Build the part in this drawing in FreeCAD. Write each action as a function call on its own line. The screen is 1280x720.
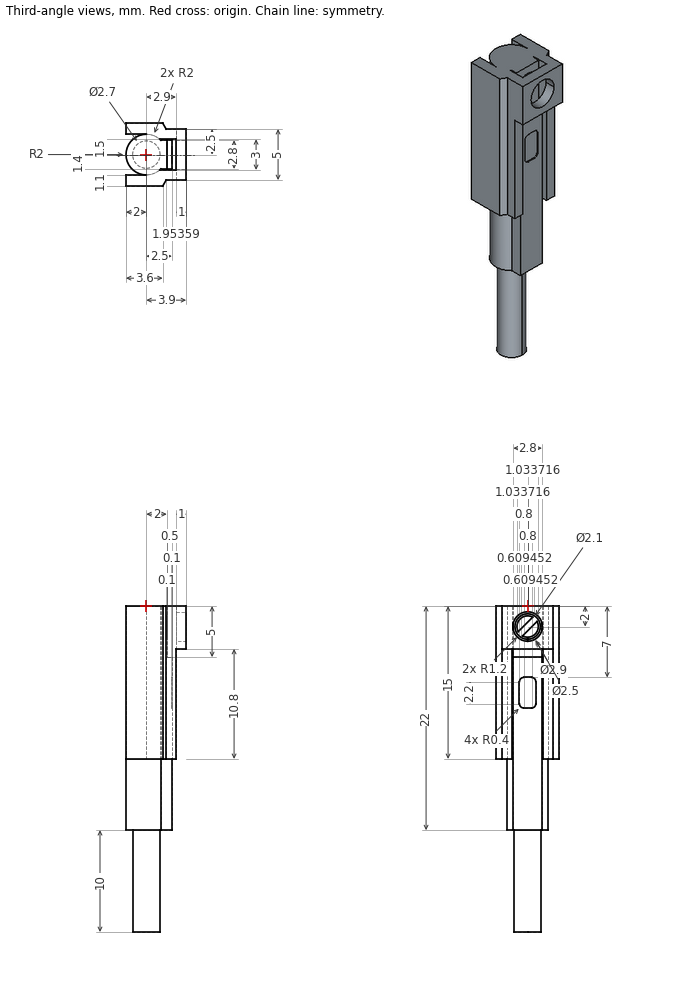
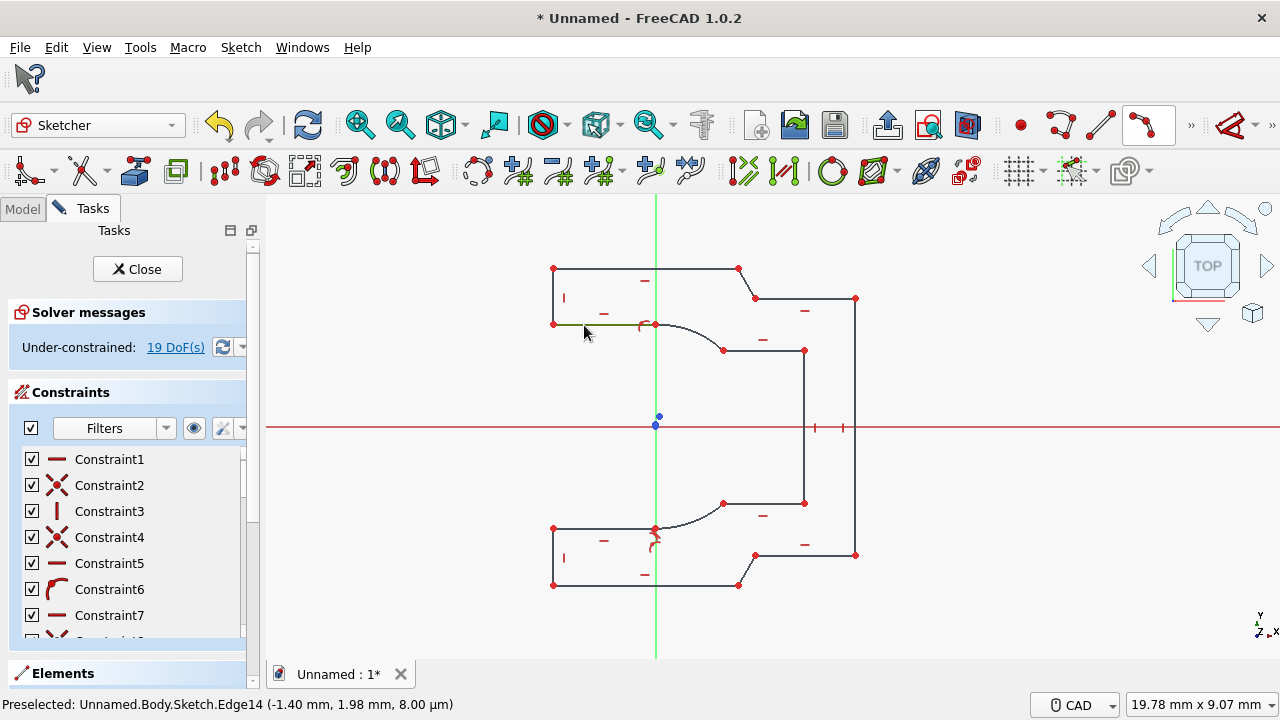
click(706, 337)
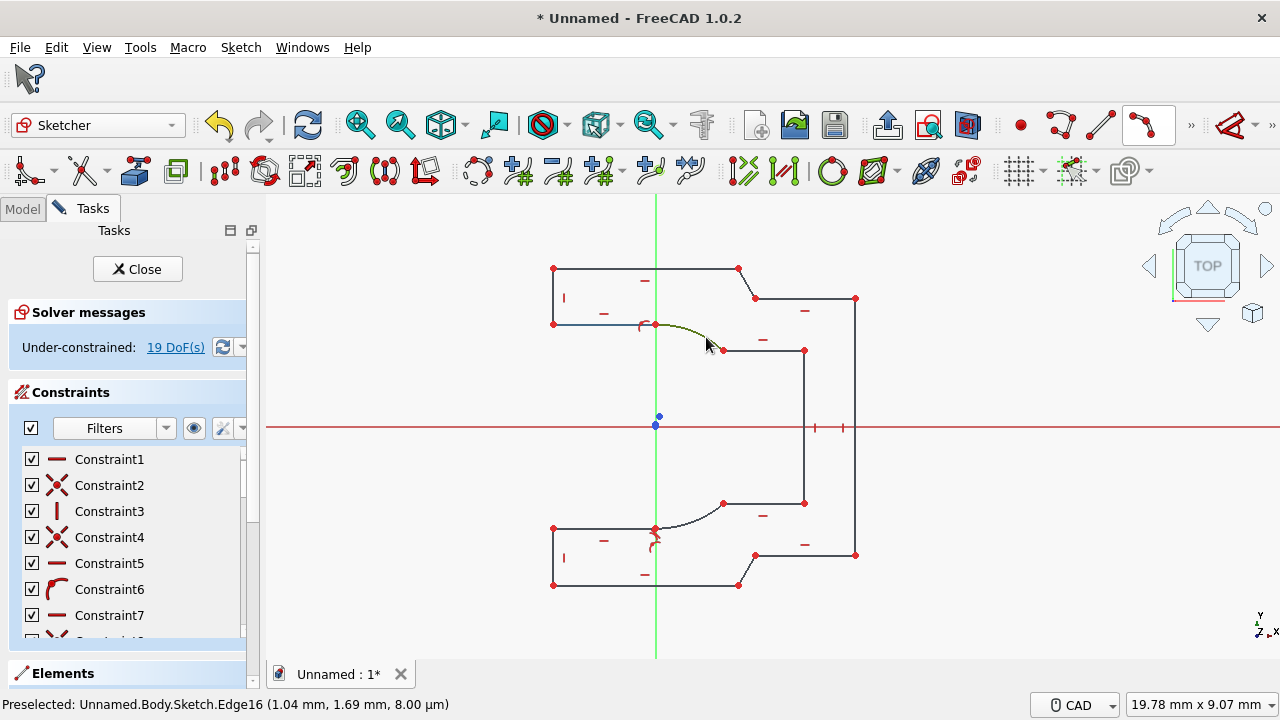
key(t)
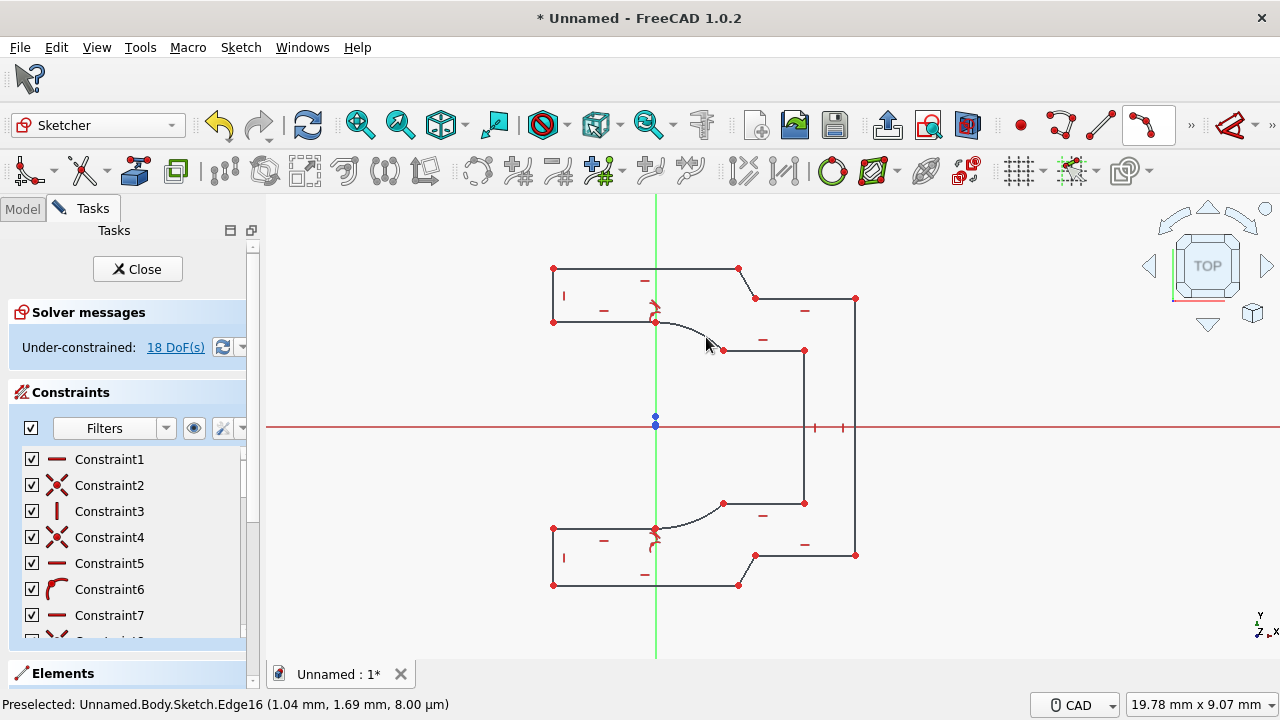
click(678, 526)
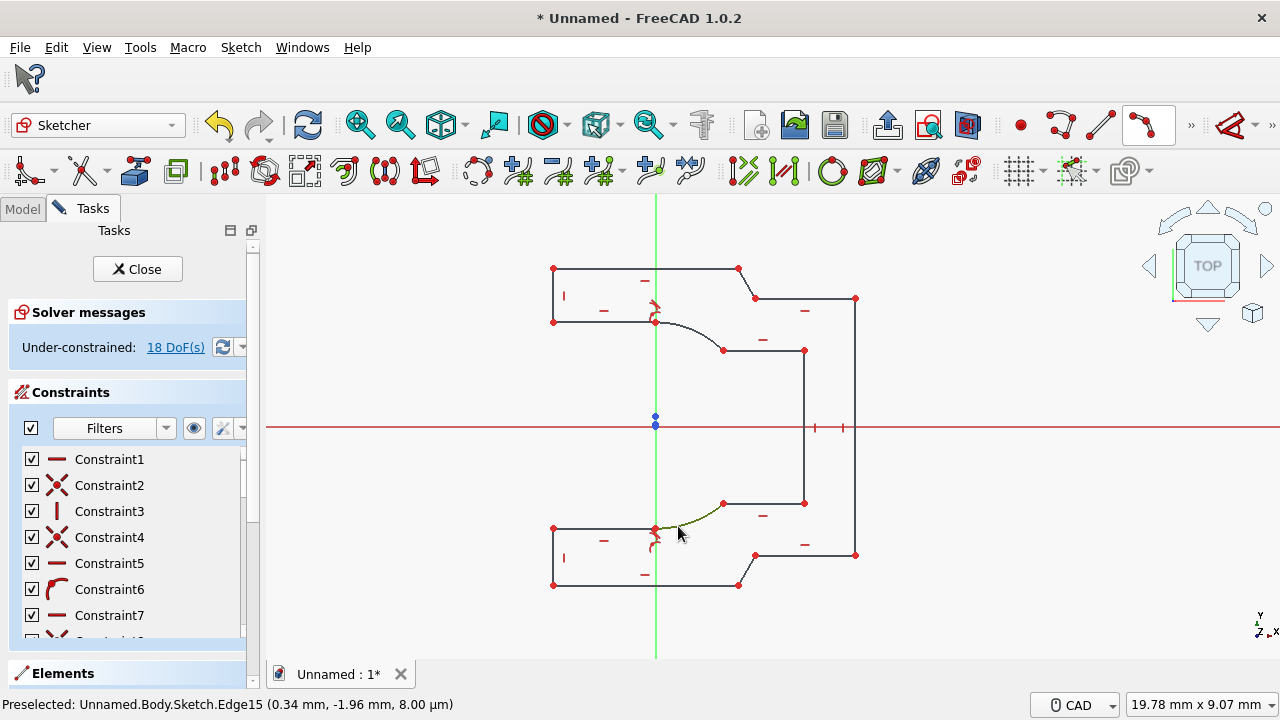
click(706, 337)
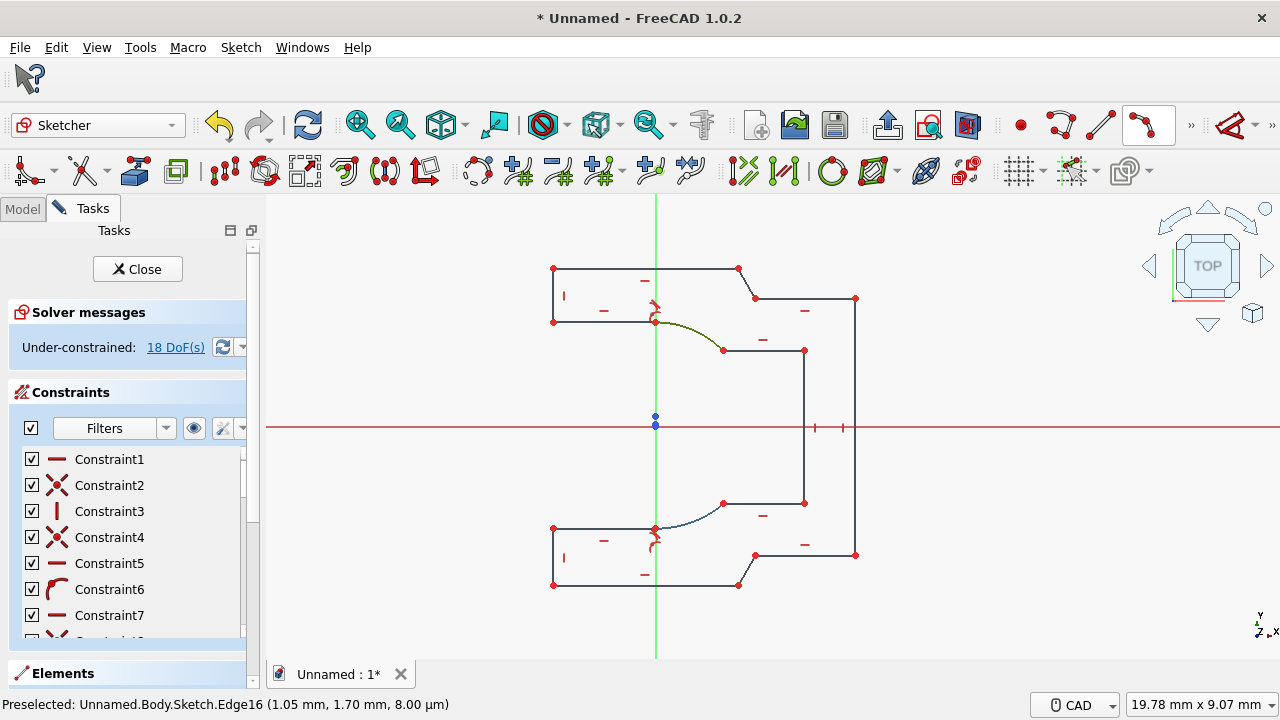
key(e)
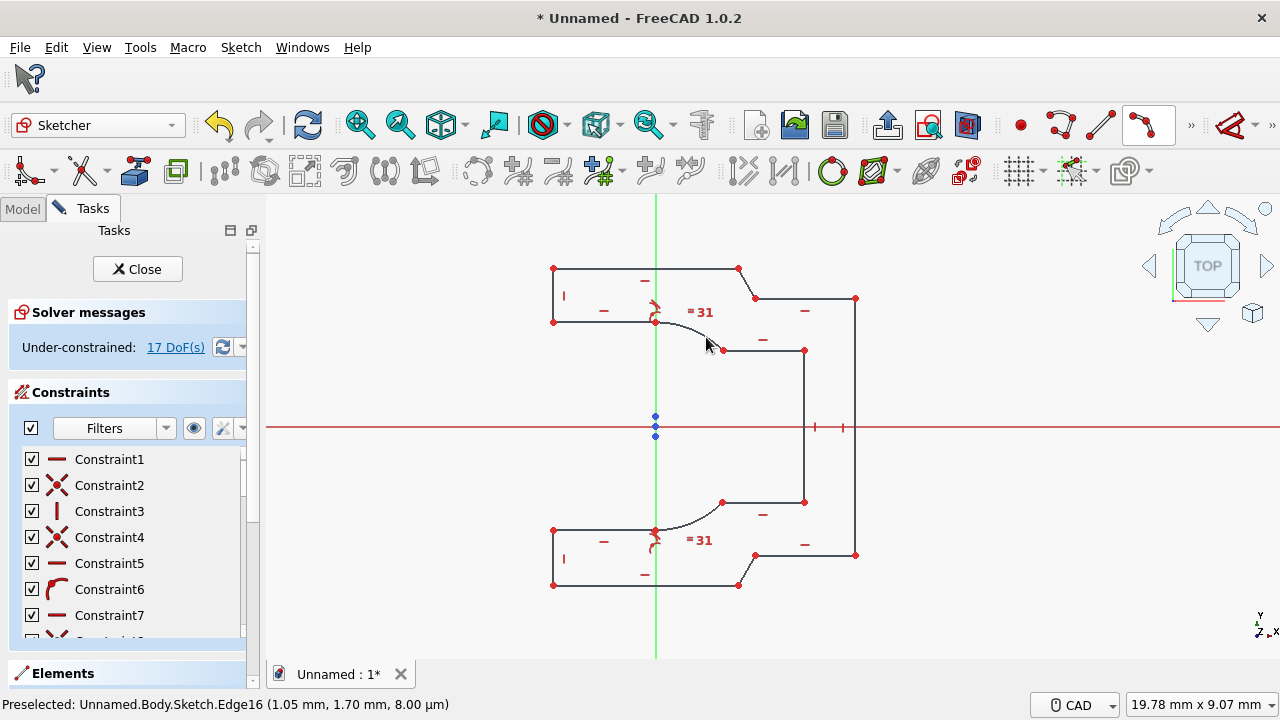
click(656, 436)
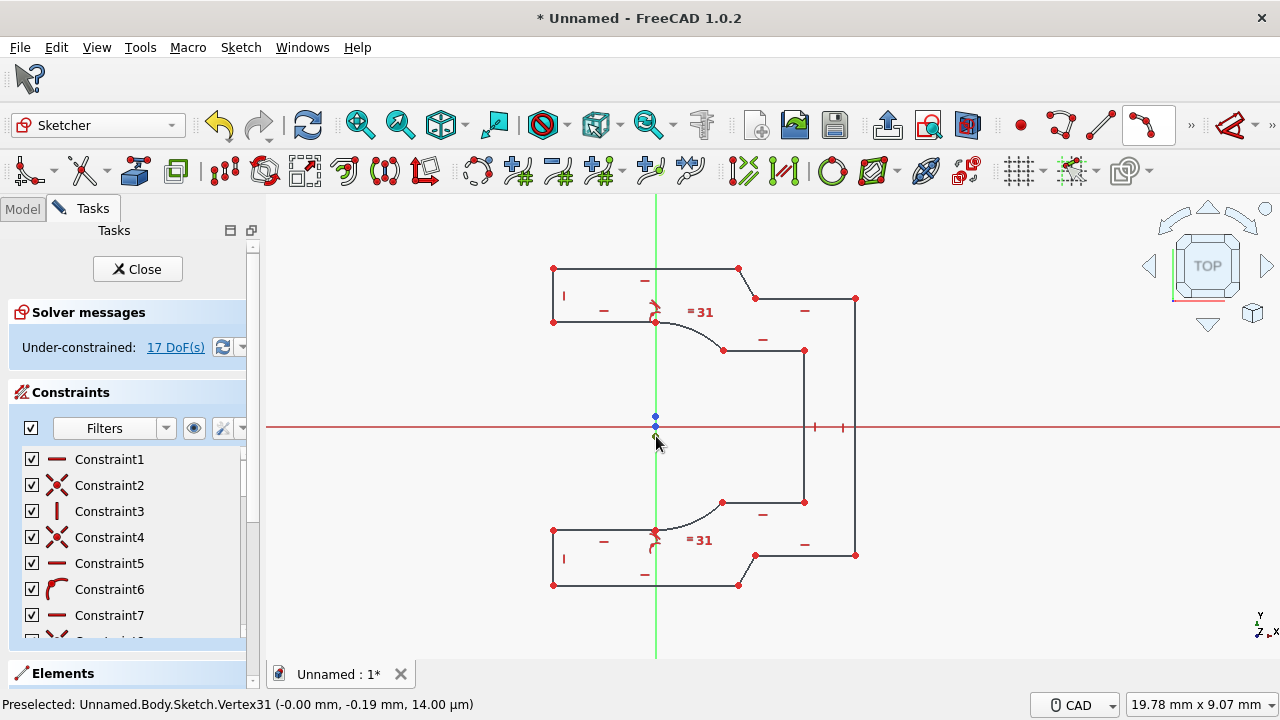
click(353, 426)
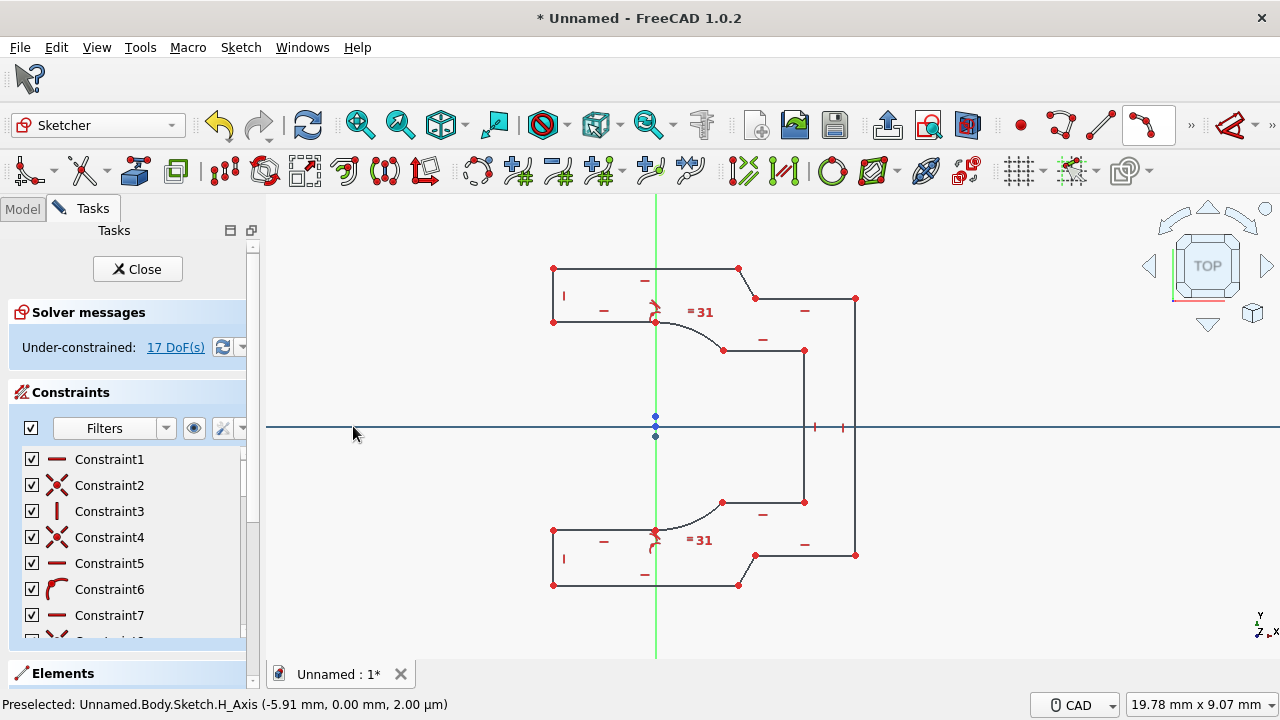
key(c)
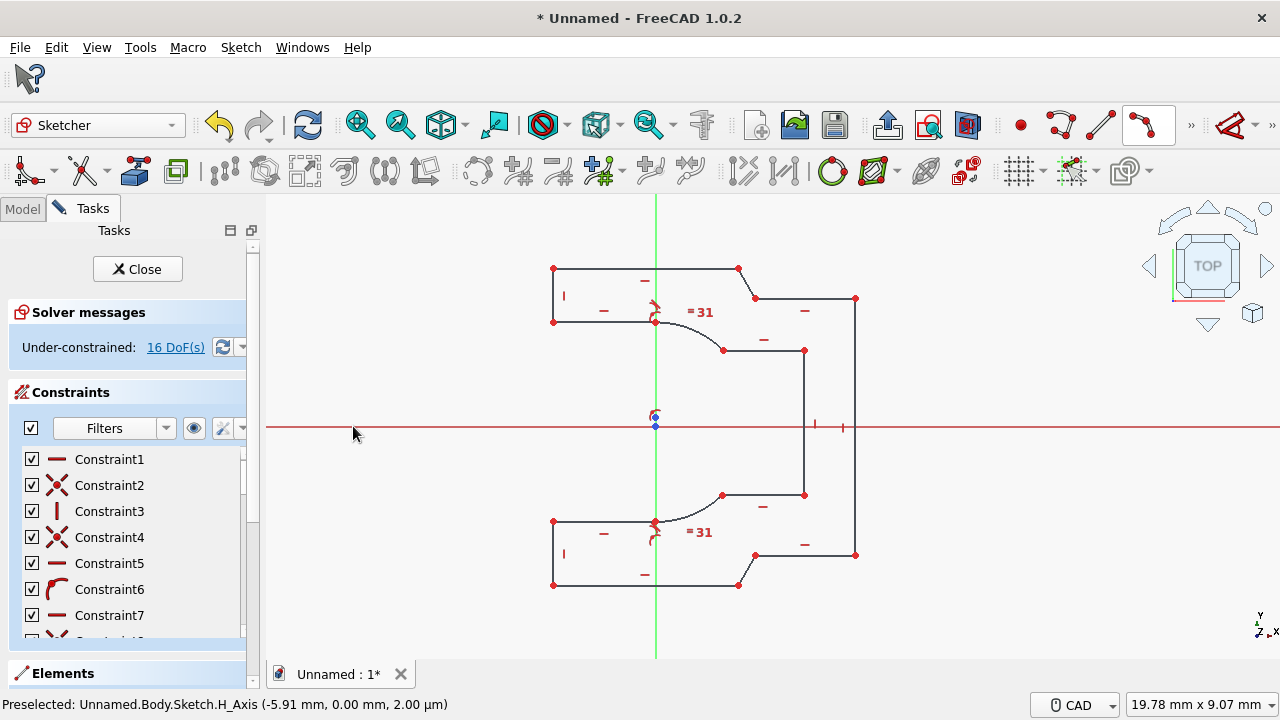
click(656, 418)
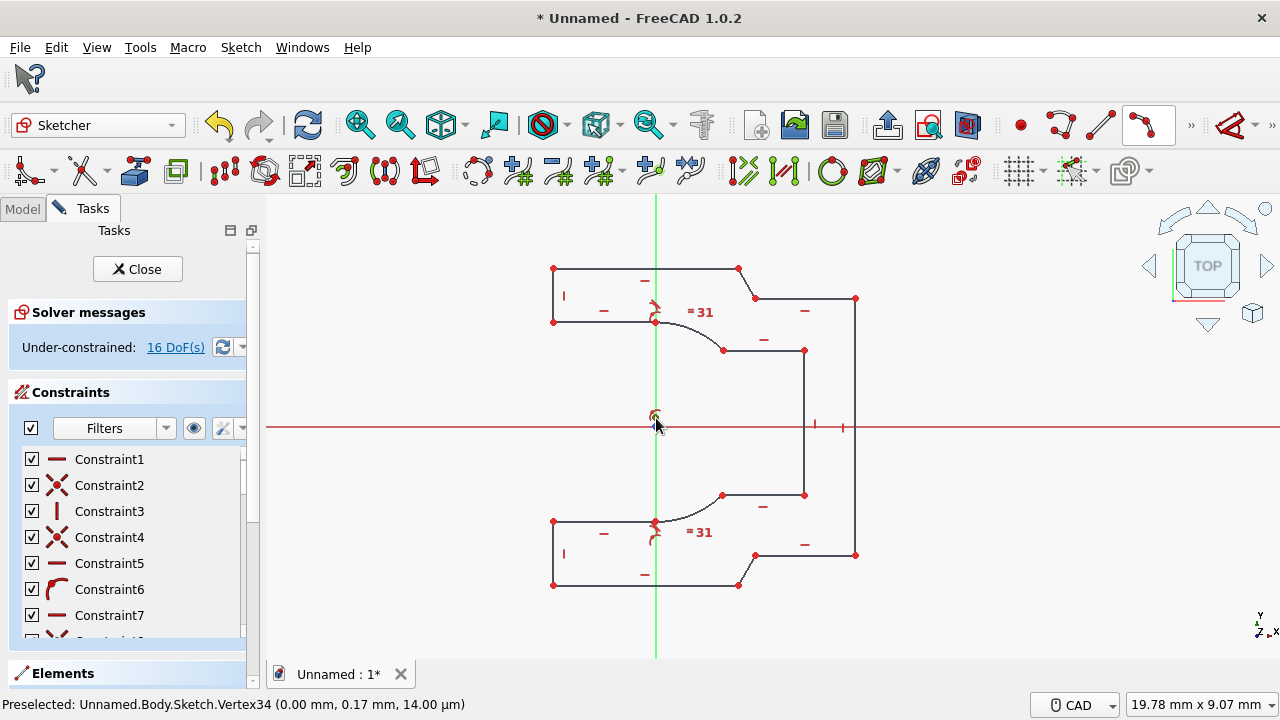
click(353, 426)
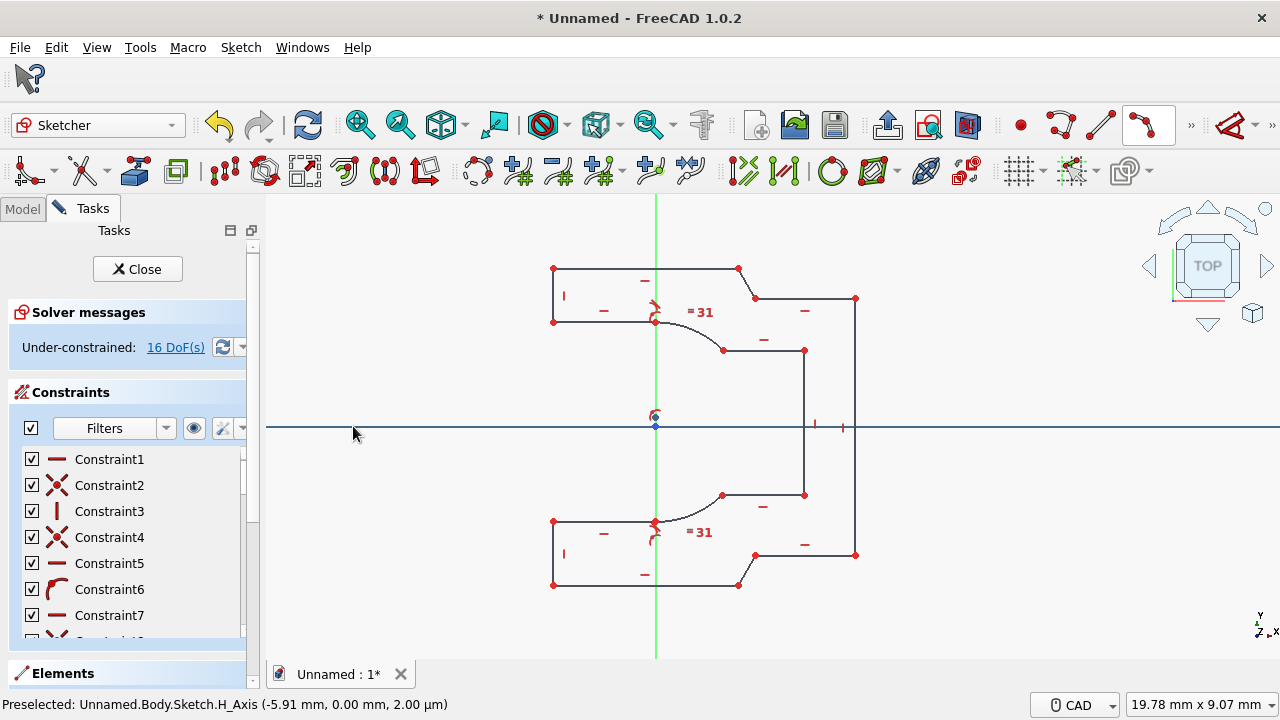
key(c)